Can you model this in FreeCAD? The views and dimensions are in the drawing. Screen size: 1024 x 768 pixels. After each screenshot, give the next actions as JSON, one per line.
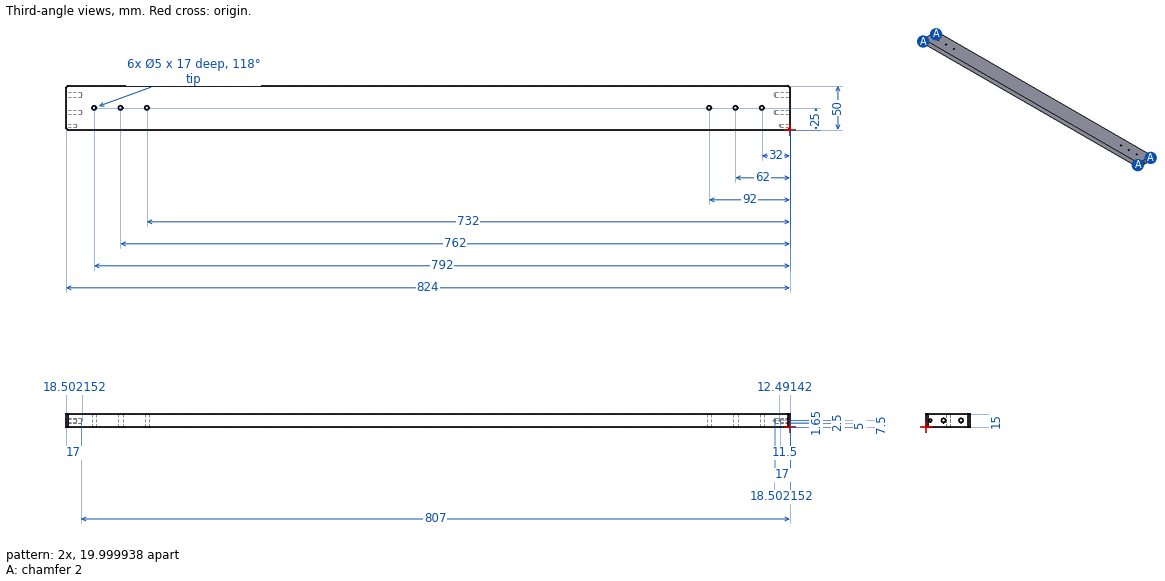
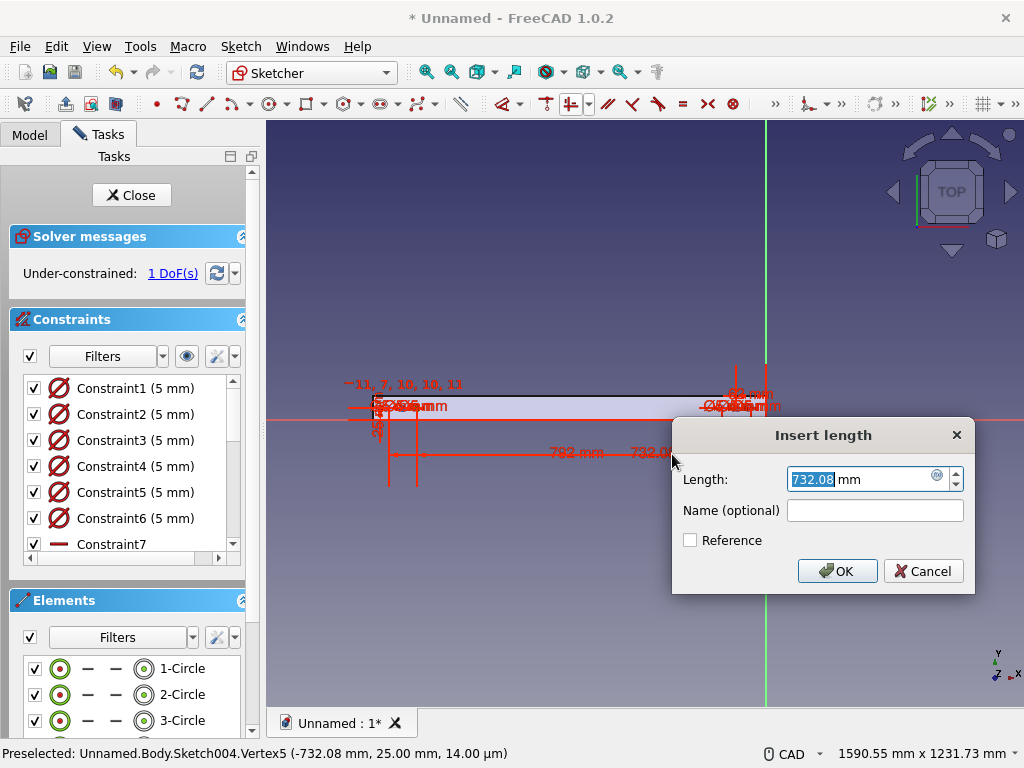
{"action": "type", "text": "732"}
{"action": "key", "text": "Return"}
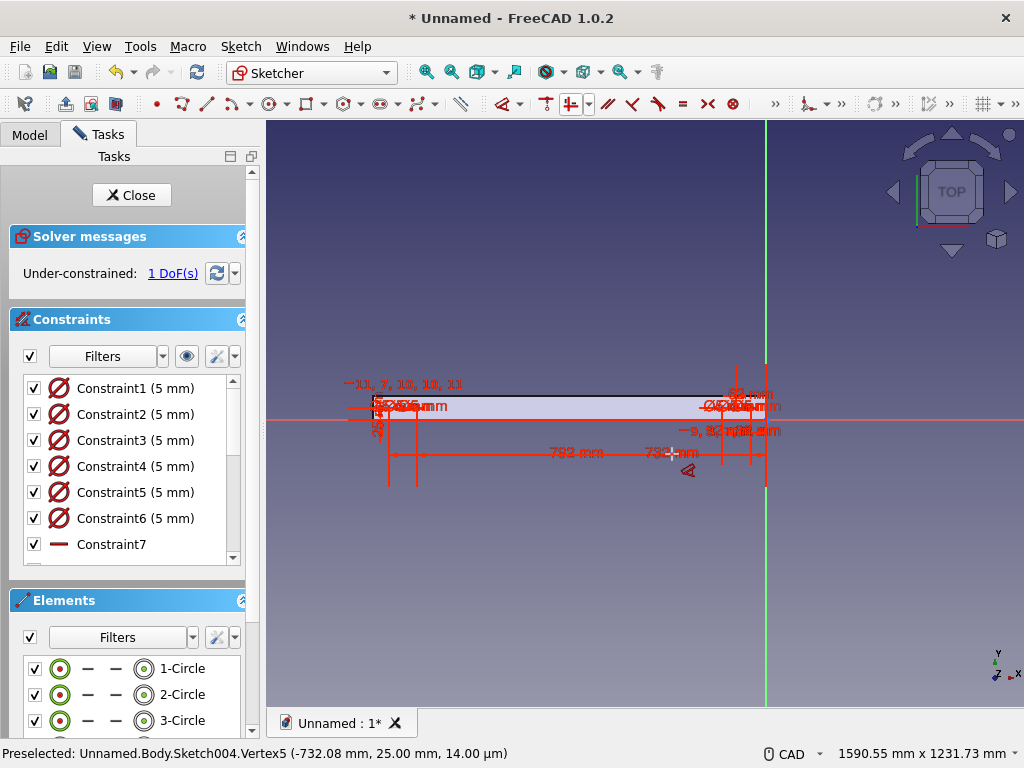
{"action": "left_click", "coordinate": [403, 408]}
{"action": "left_click", "coordinate": [501, 454]}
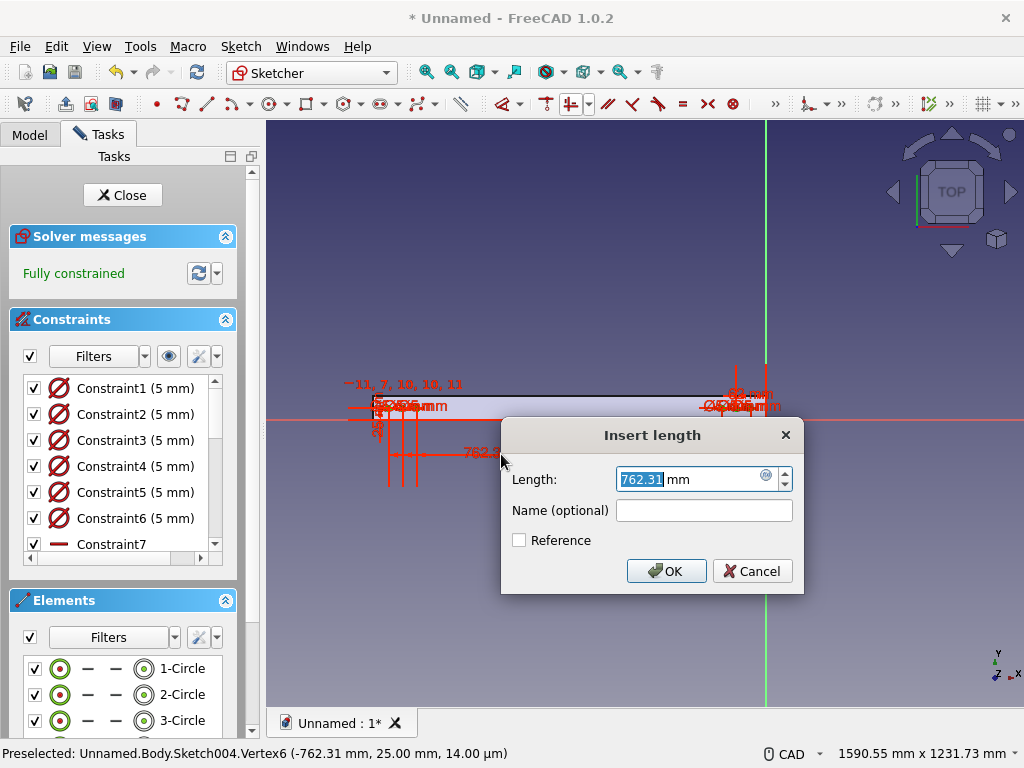
{"action": "type", "text": "762"}
{"action": "key", "text": "Return"}
{"action": "key", "text": "Escape"}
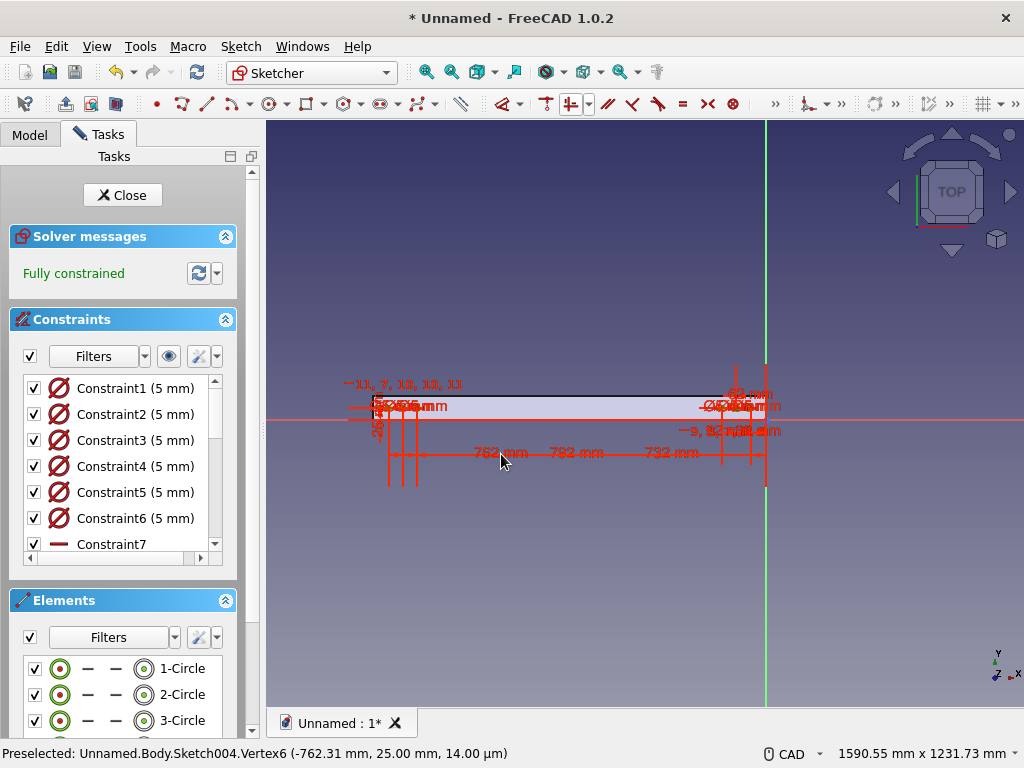
{"action": "left_click", "coordinate": [123, 195]}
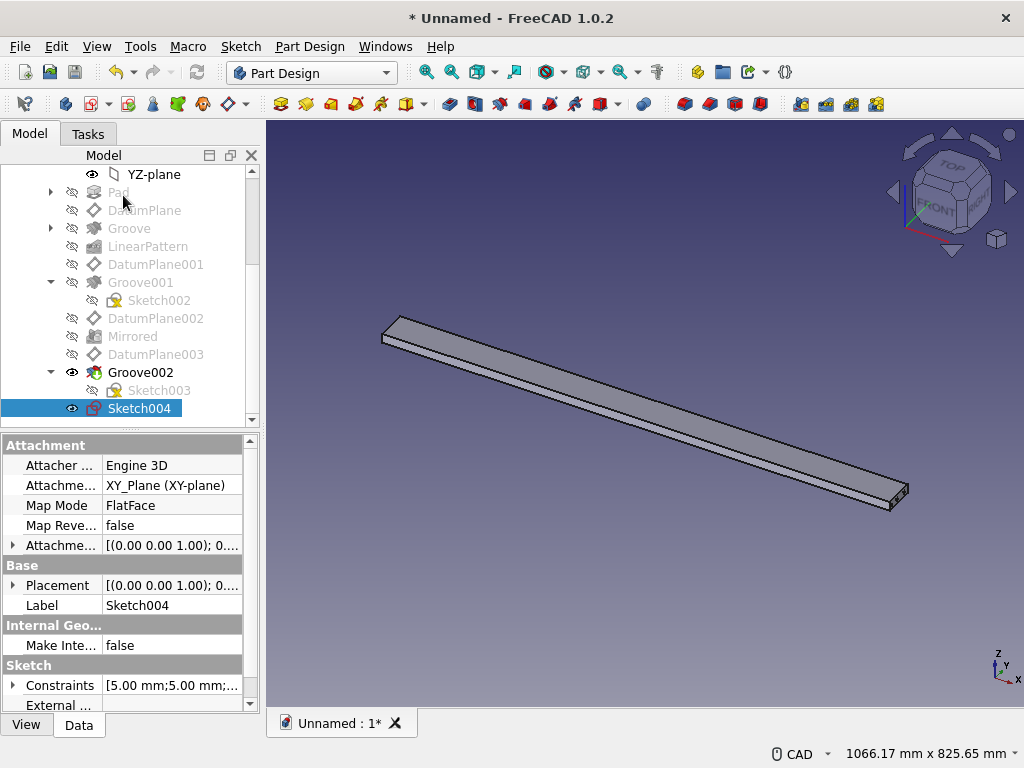
{"action": "left_click", "coordinate": [475, 104]}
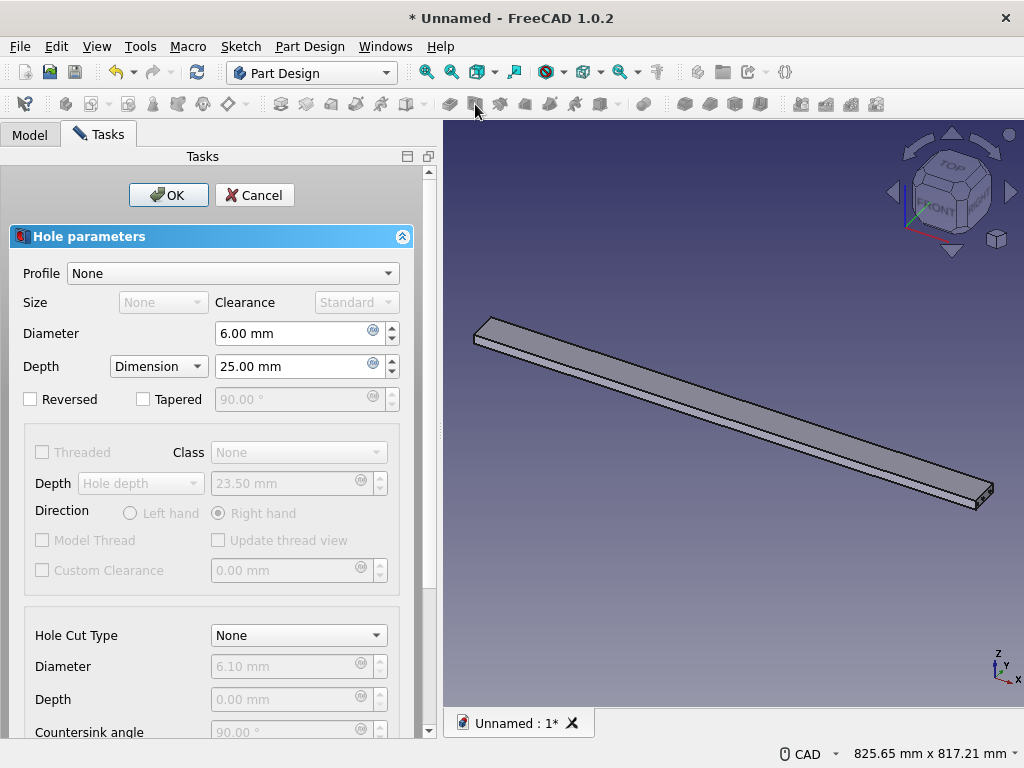
{"action": "triple_click", "coordinate": [300, 334]}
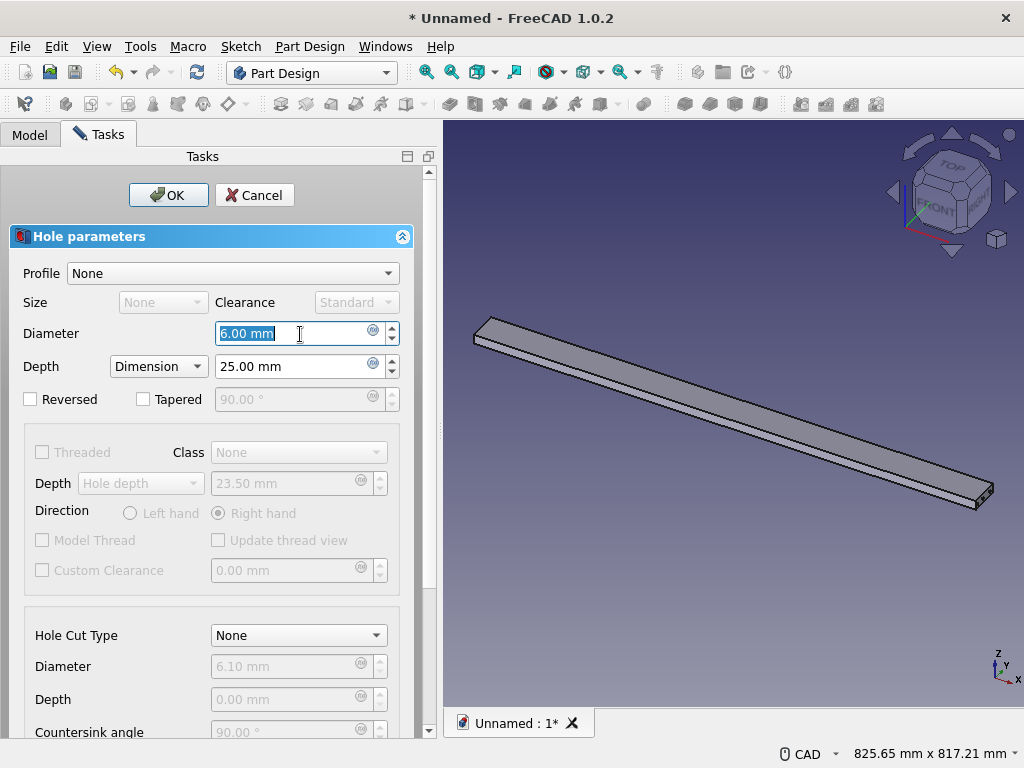
{"action": "type", "text": "5"}
{"action": "key", "text": "Tab"}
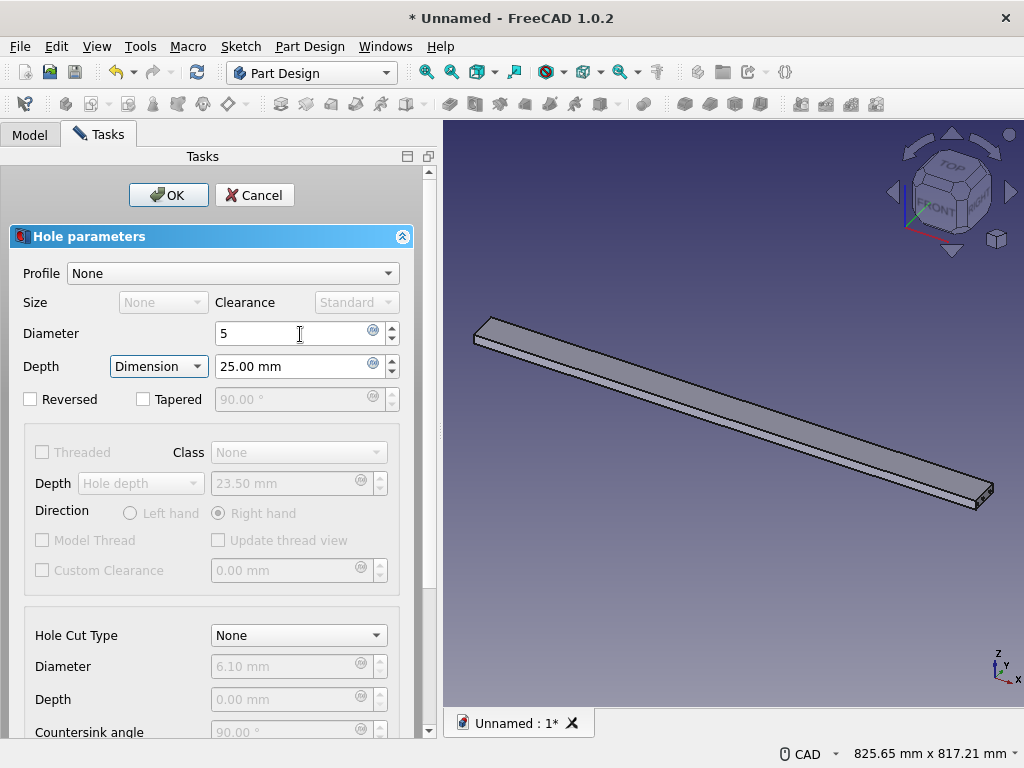
{"action": "triple_click", "coordinate": [300, 366]}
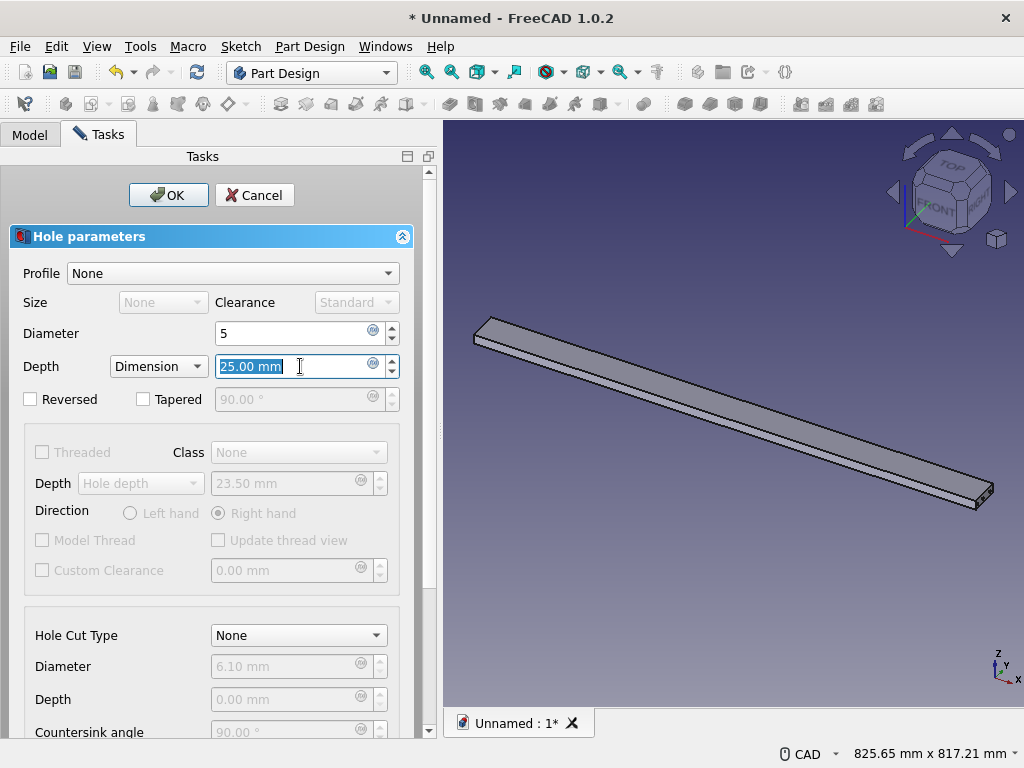
{"action": "type", "text": "17"}
{"action": "key", "text": "Tab"}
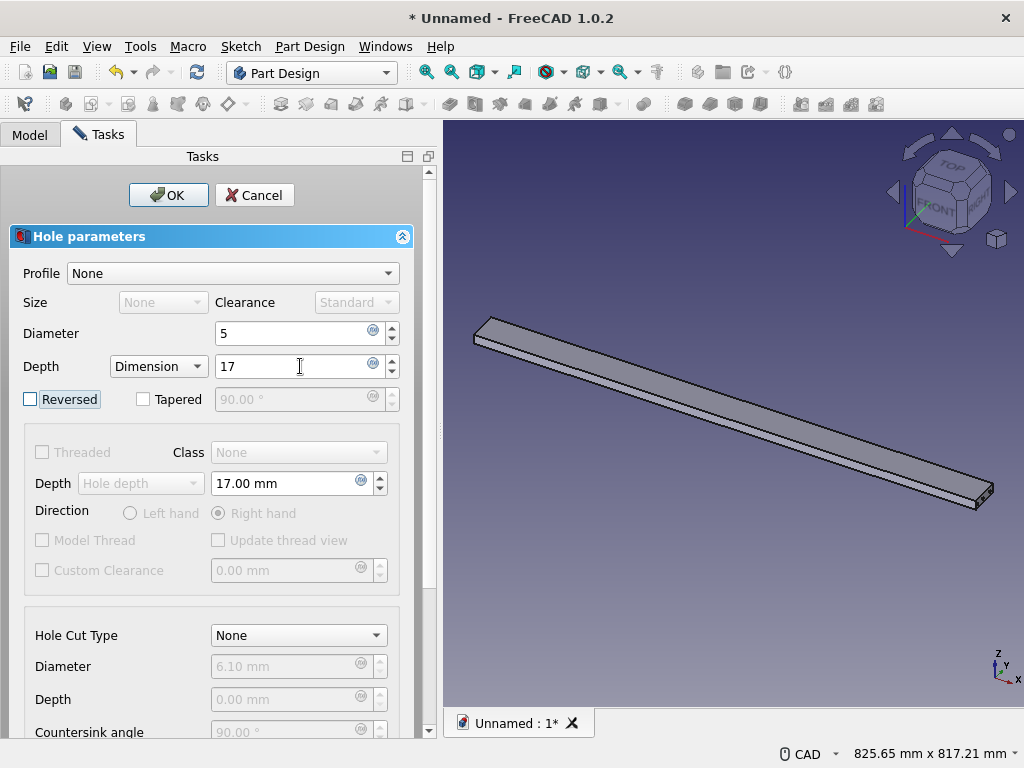
{"action": "left_click", "coordinate": [31, 399]}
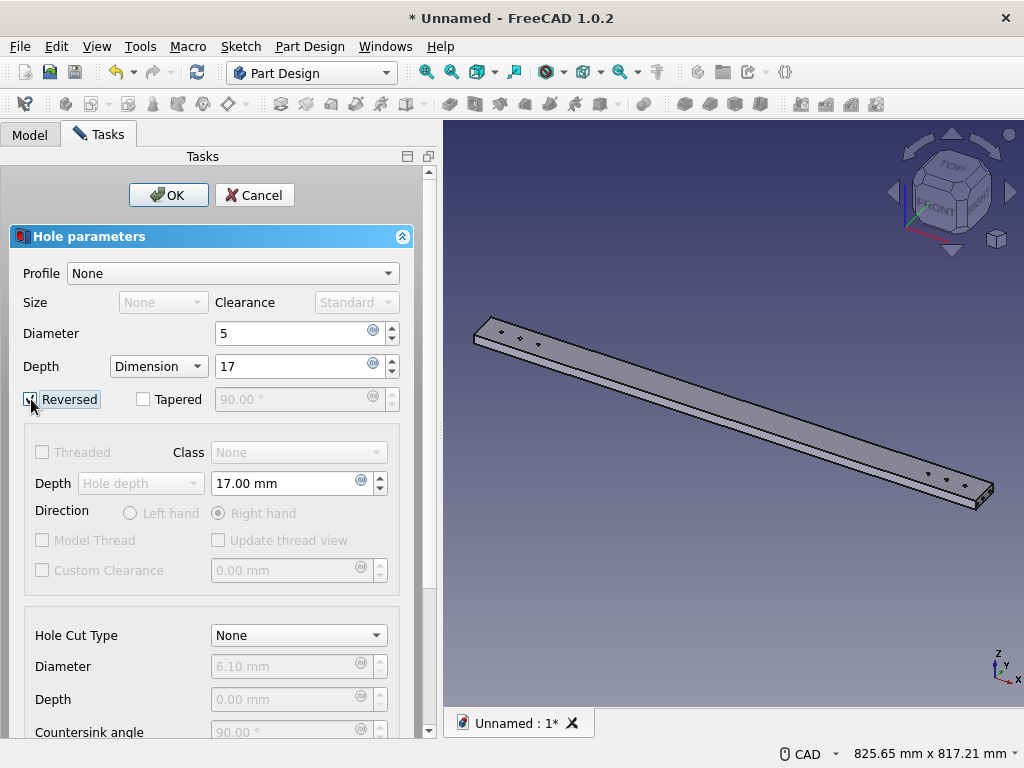
{"action": "left_click", "coordinate": [169, 195]}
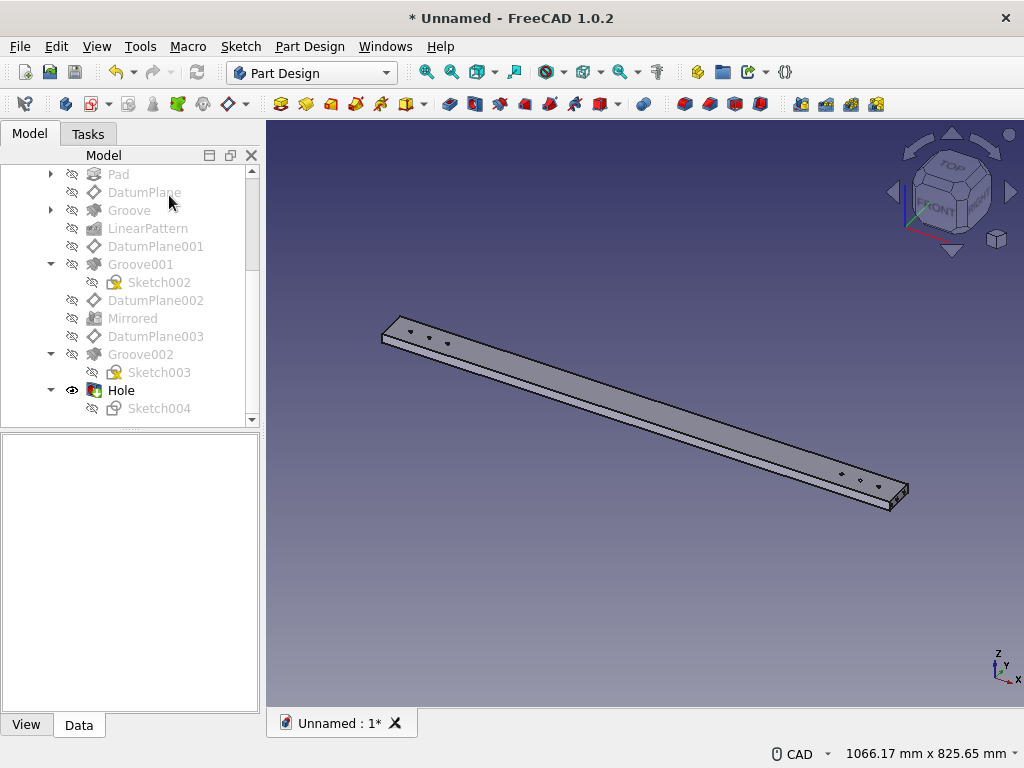
{"action": "key", "text": "0"}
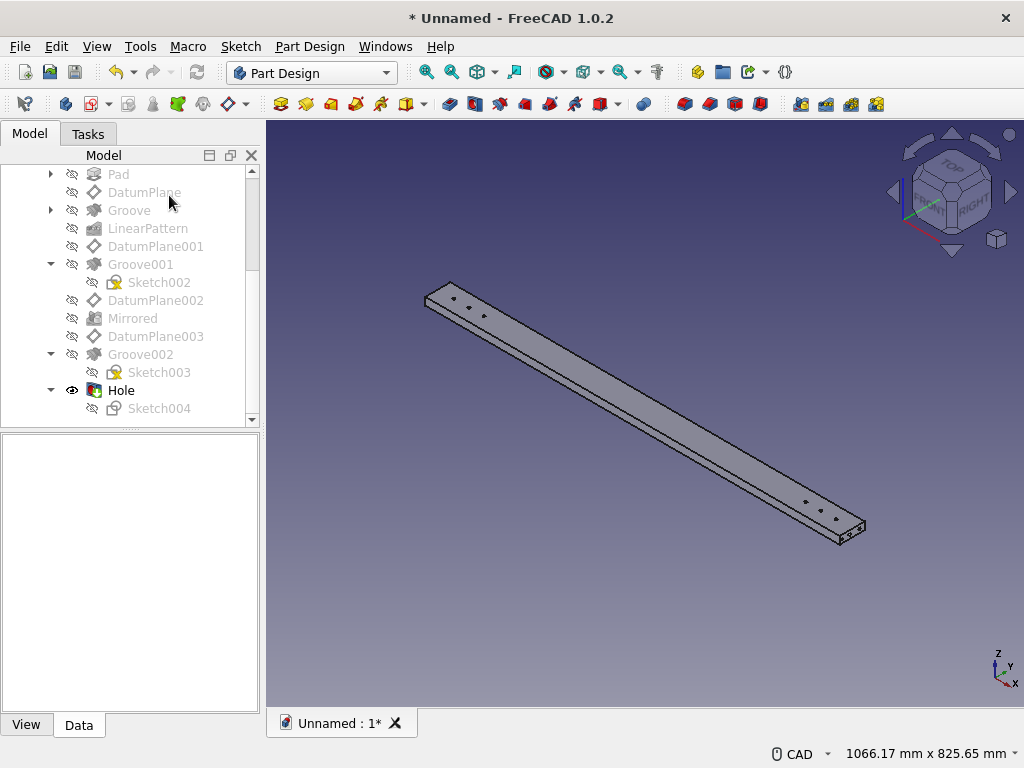
{"action": "key", "text": "2"}